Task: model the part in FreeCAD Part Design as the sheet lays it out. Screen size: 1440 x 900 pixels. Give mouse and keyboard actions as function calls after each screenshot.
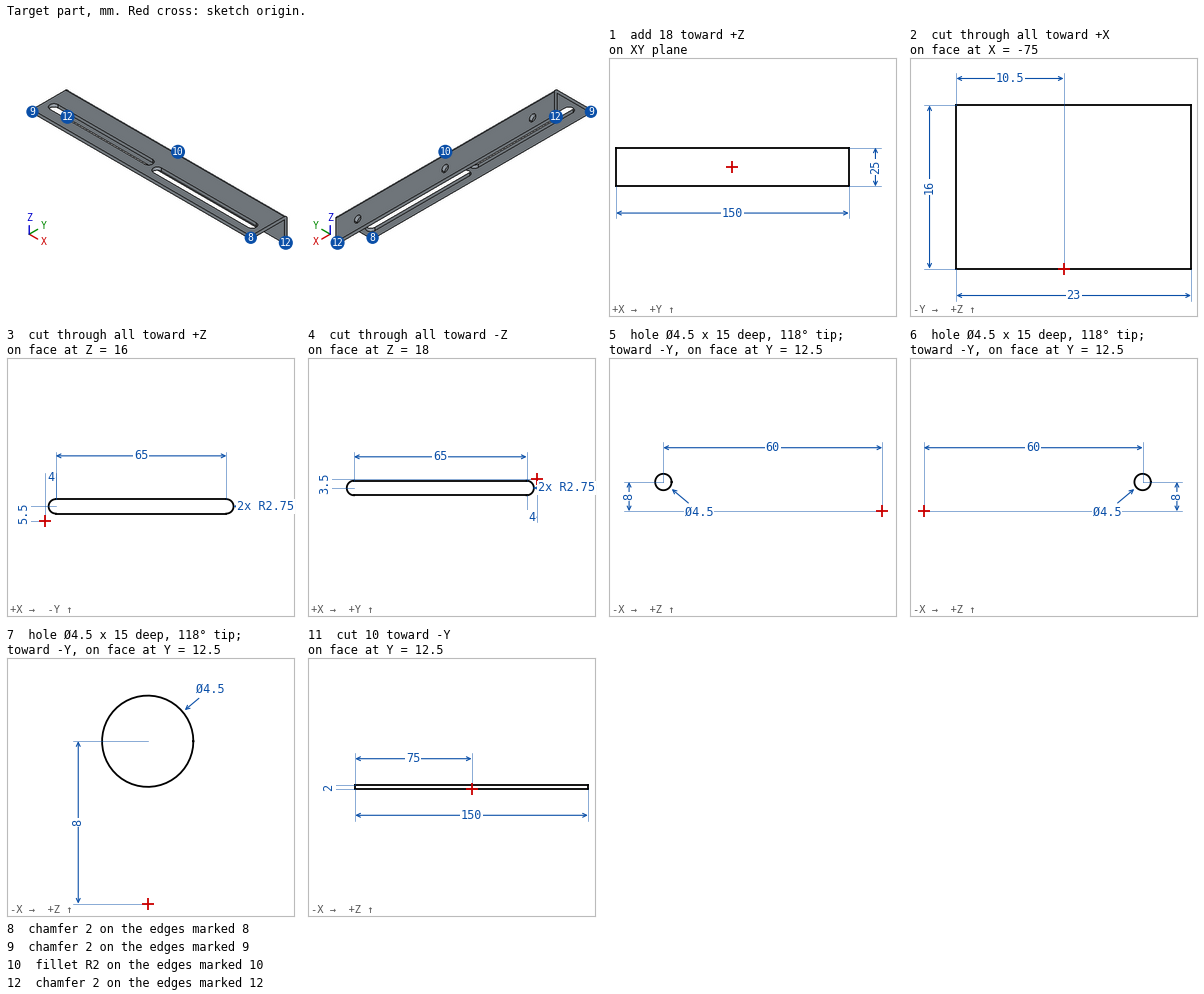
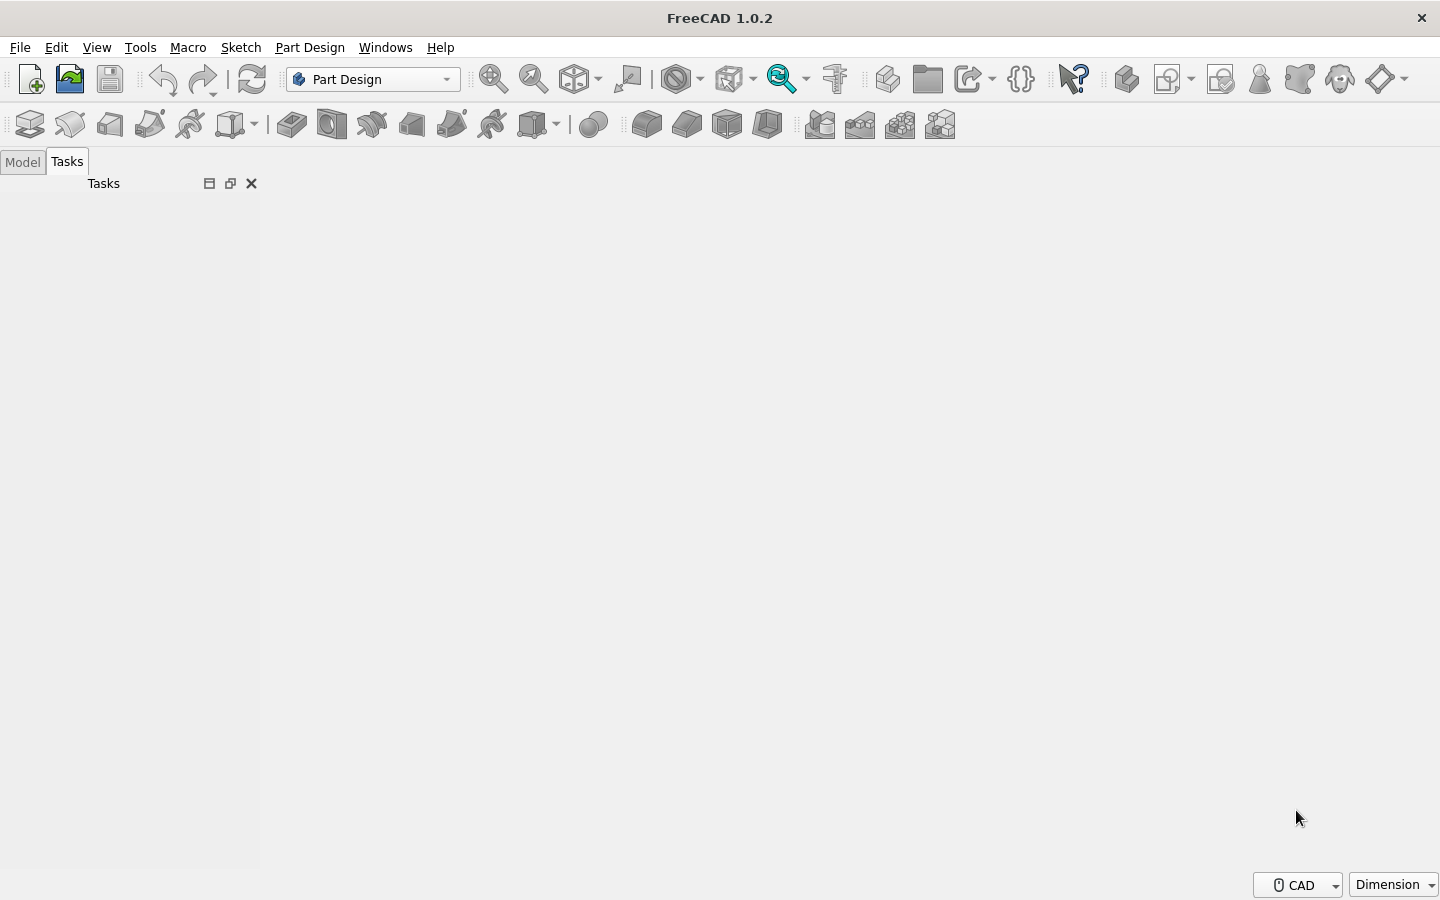
click(30, 80)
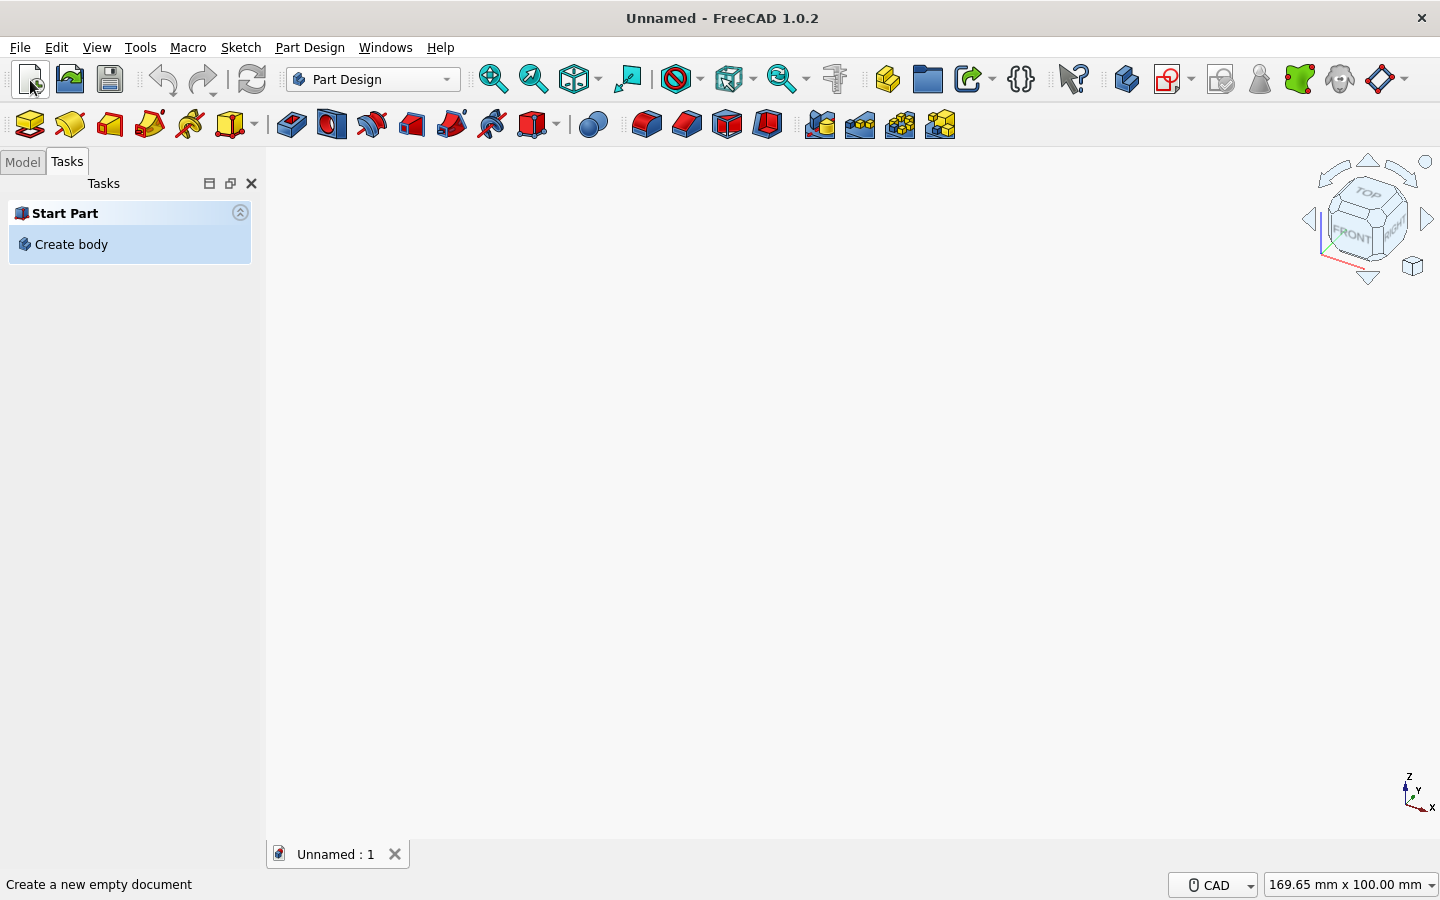
click(1168, 80)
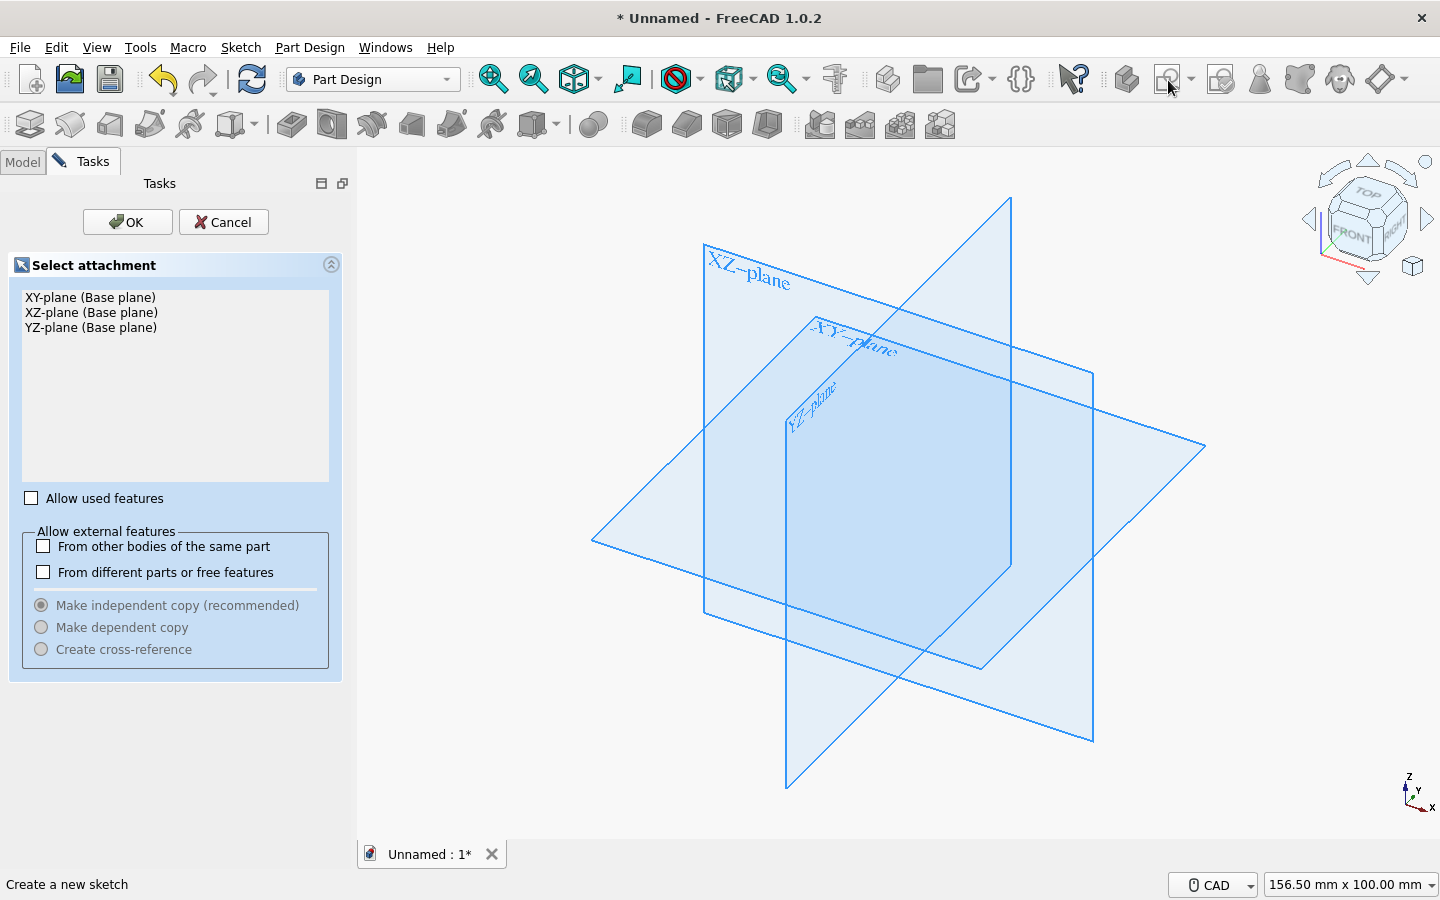
click(82, 298)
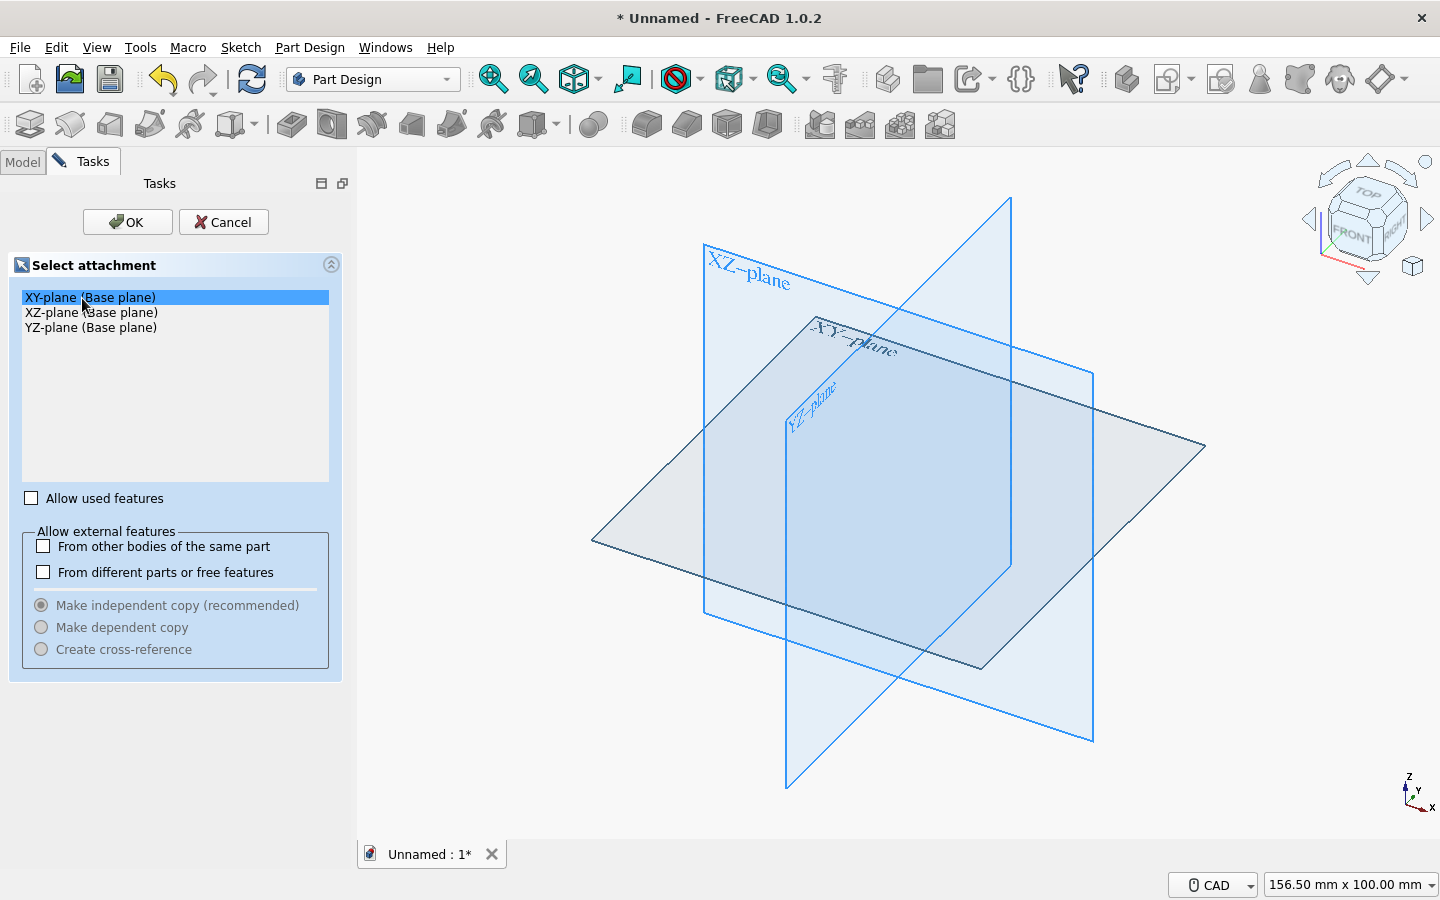
click(128, 222)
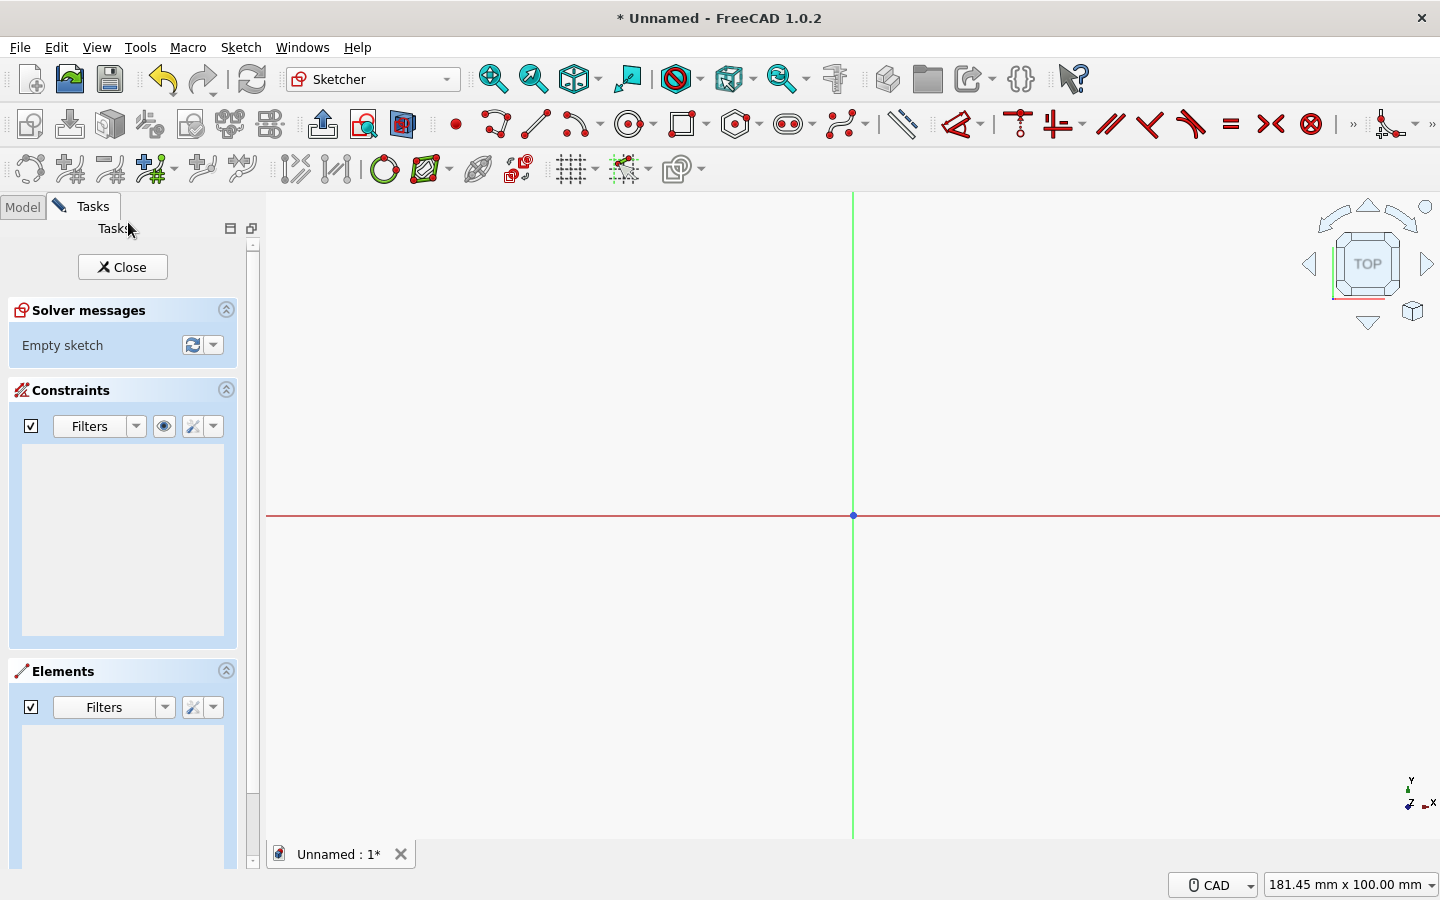
scroll(645, 515, down, 2)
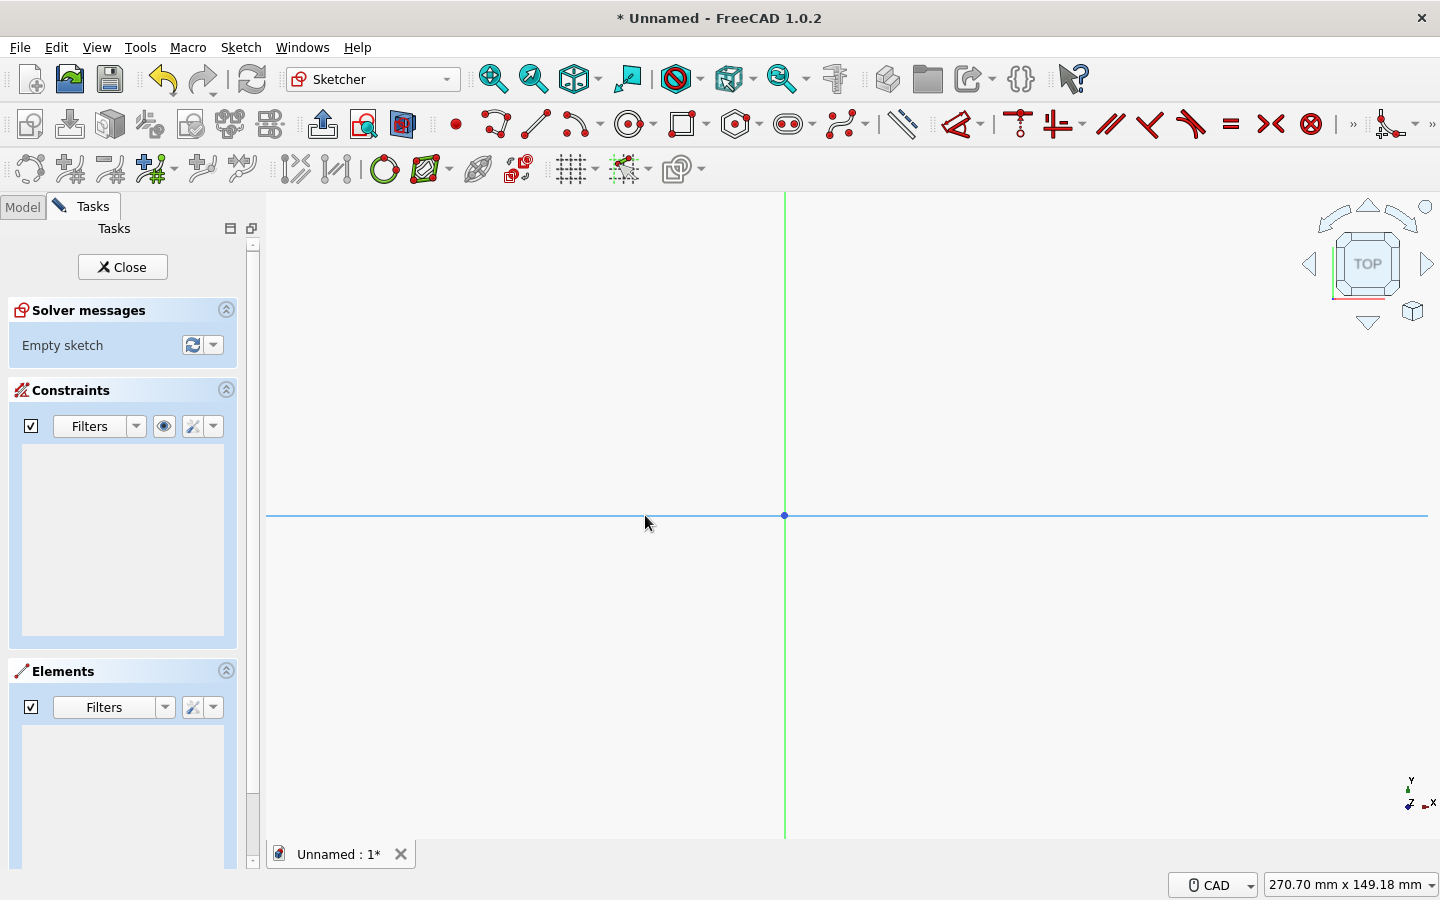
key(g)
key(v)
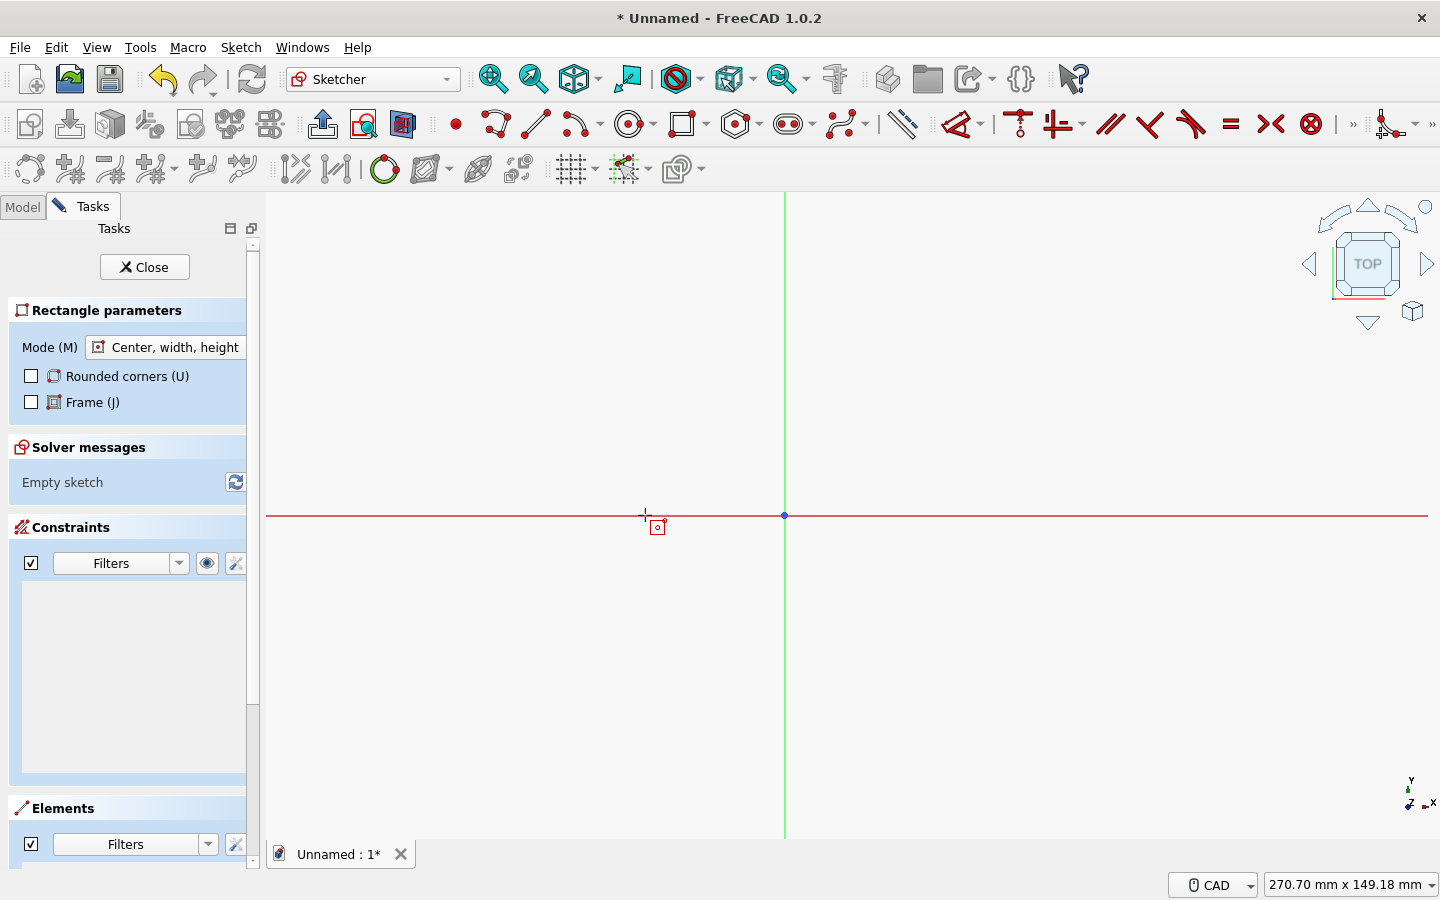
click(785, 516)
move(1110, 461)